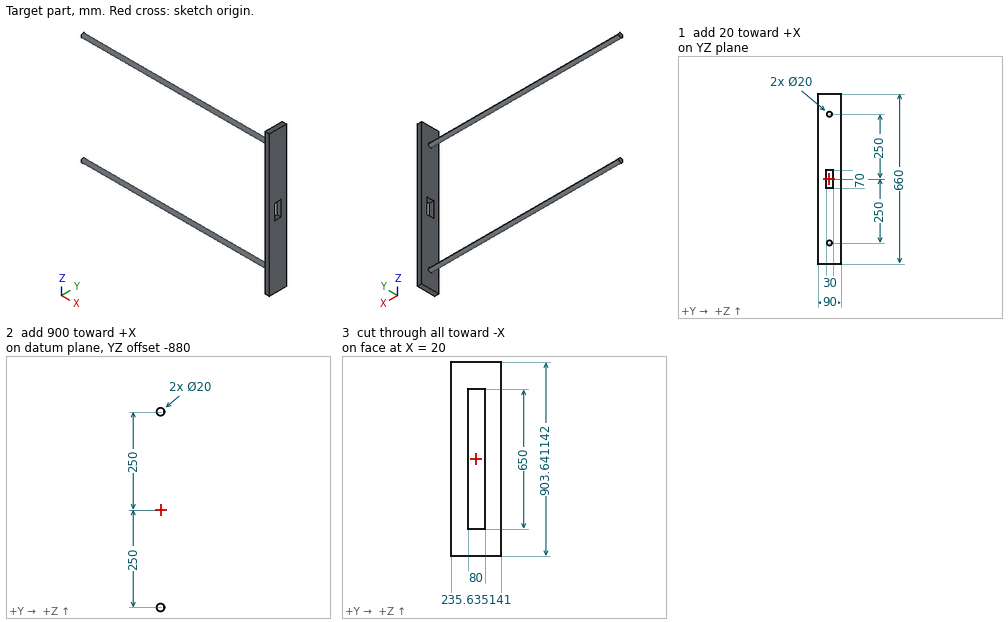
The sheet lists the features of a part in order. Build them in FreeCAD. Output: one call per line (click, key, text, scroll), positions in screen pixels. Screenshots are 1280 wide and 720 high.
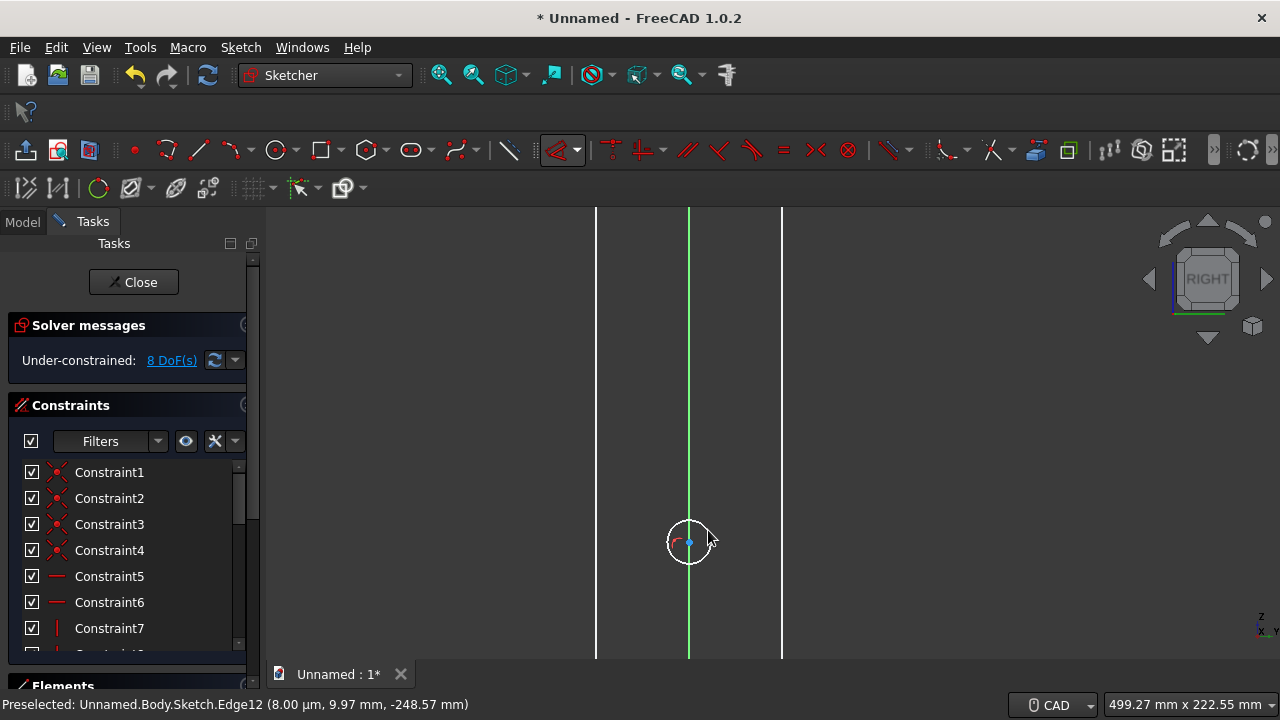
scroll(708, 535, down, 8)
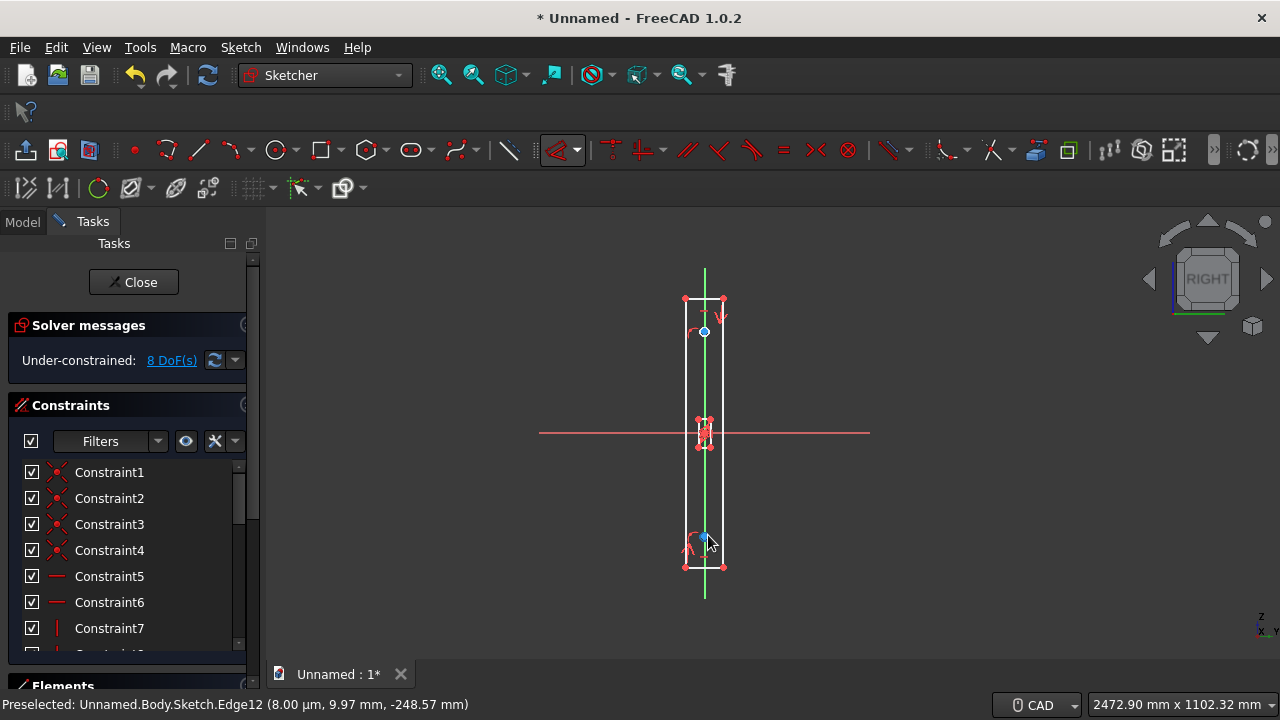
scroll(708, 329, up, 8)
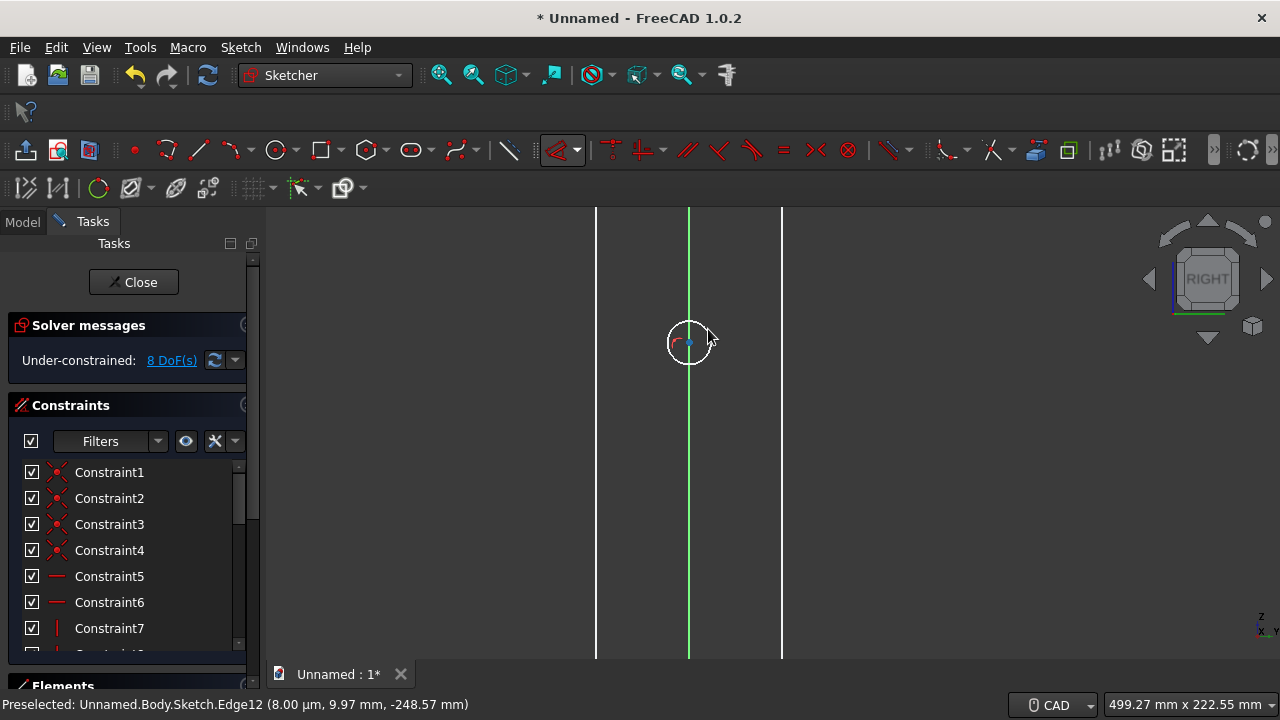
click(705, 327)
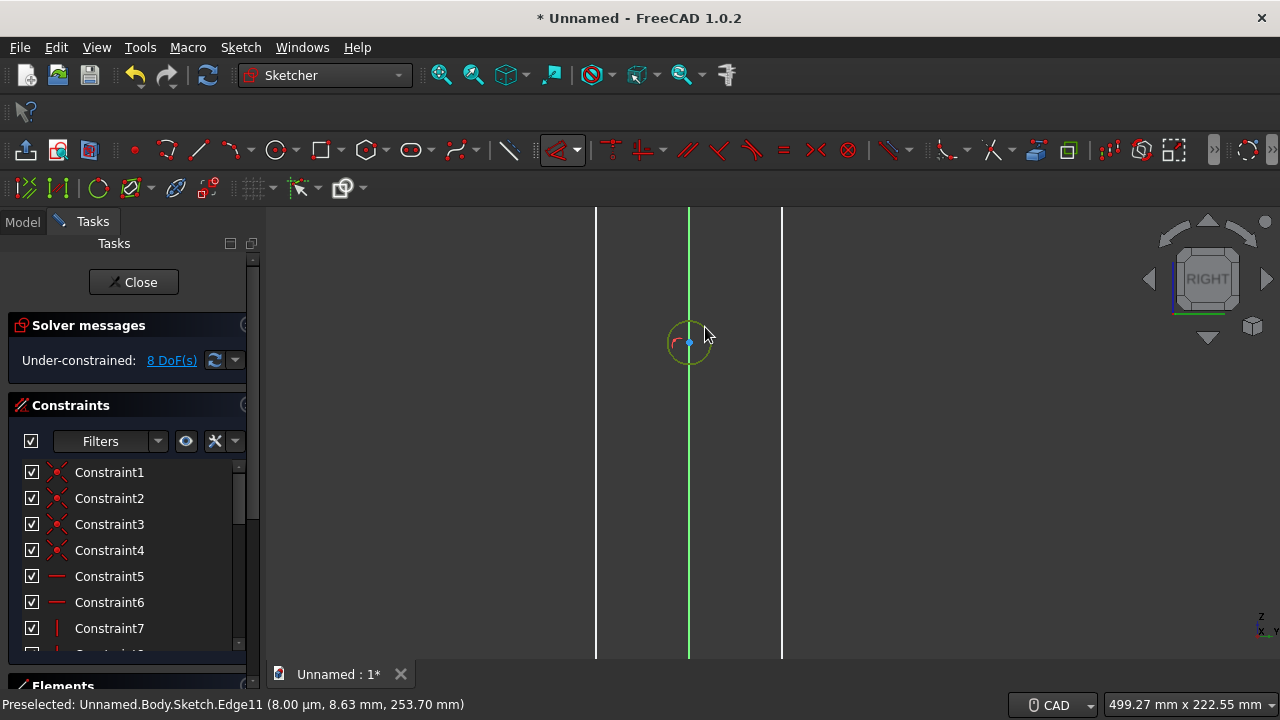
scroll(708, 329, down, 8)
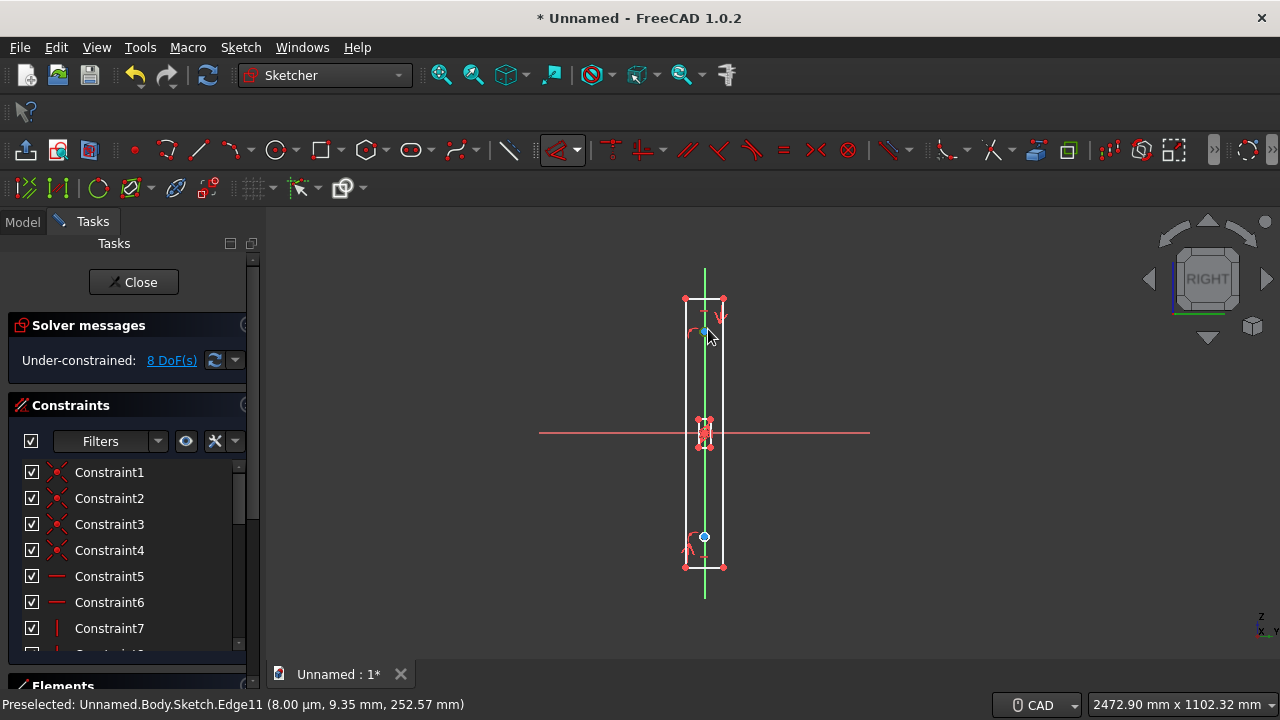
scroll(708, 534, up, 8)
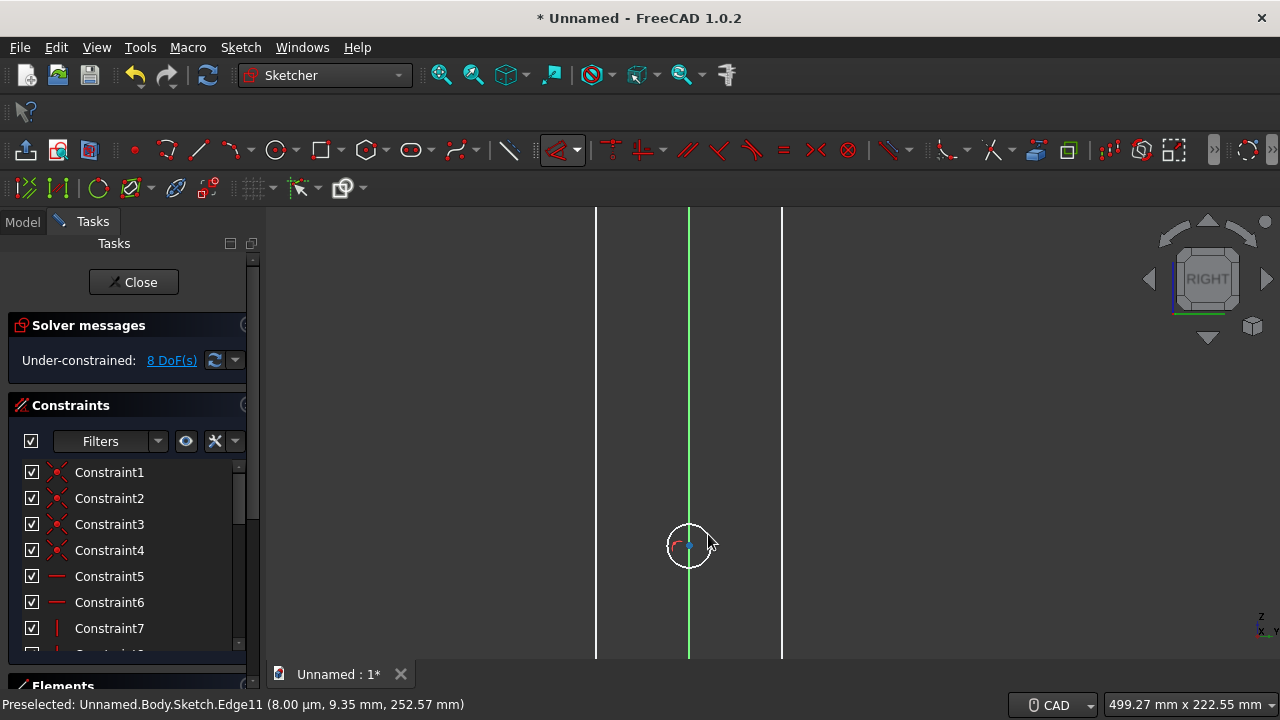
click(705, 531)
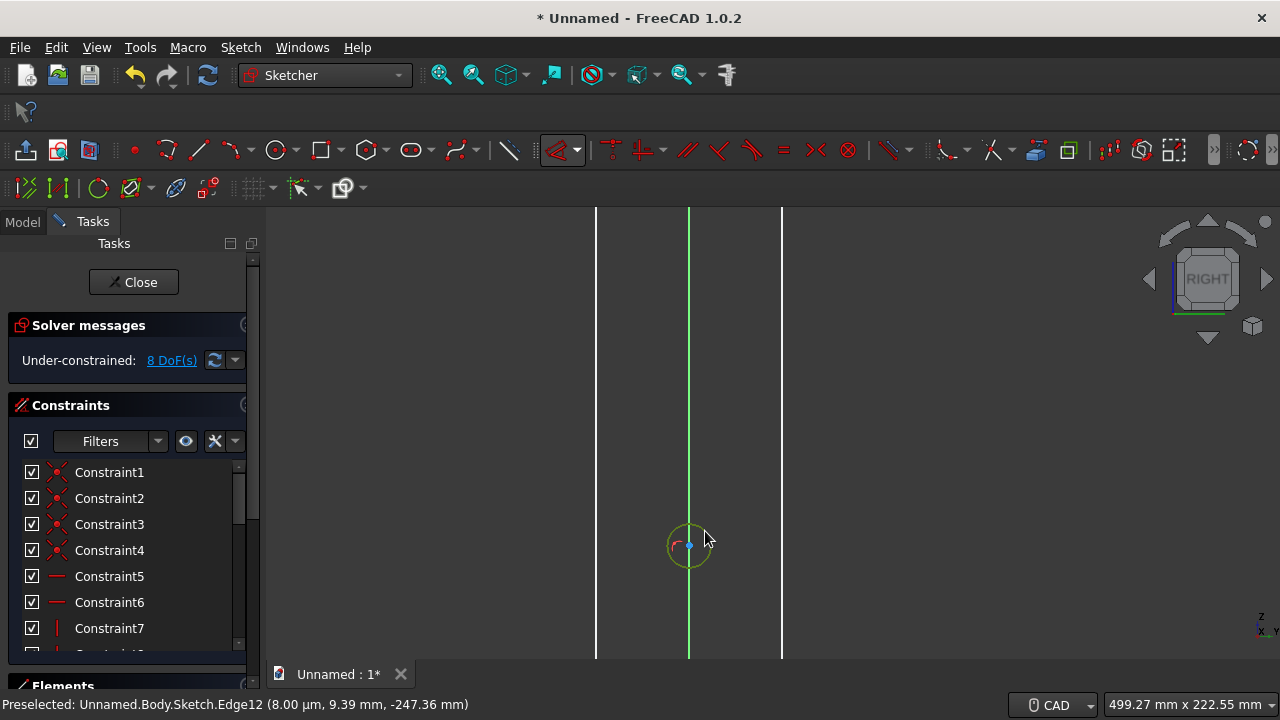
key(e)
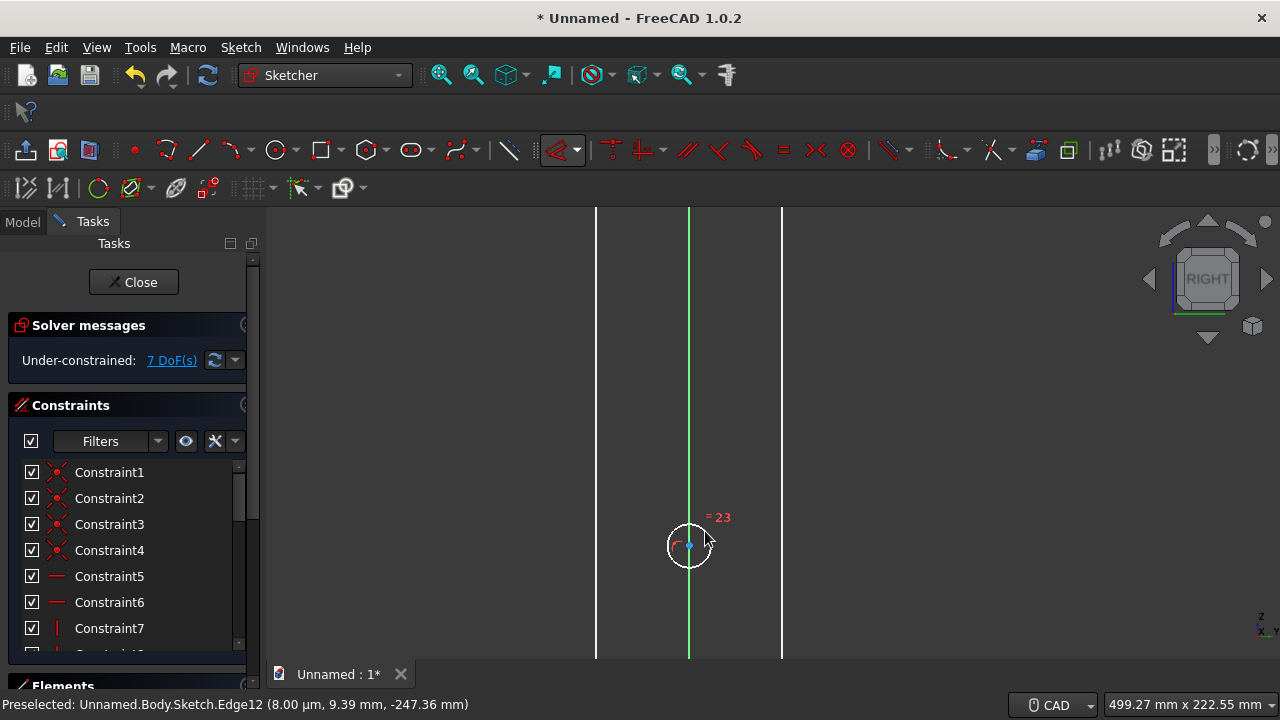
key(d)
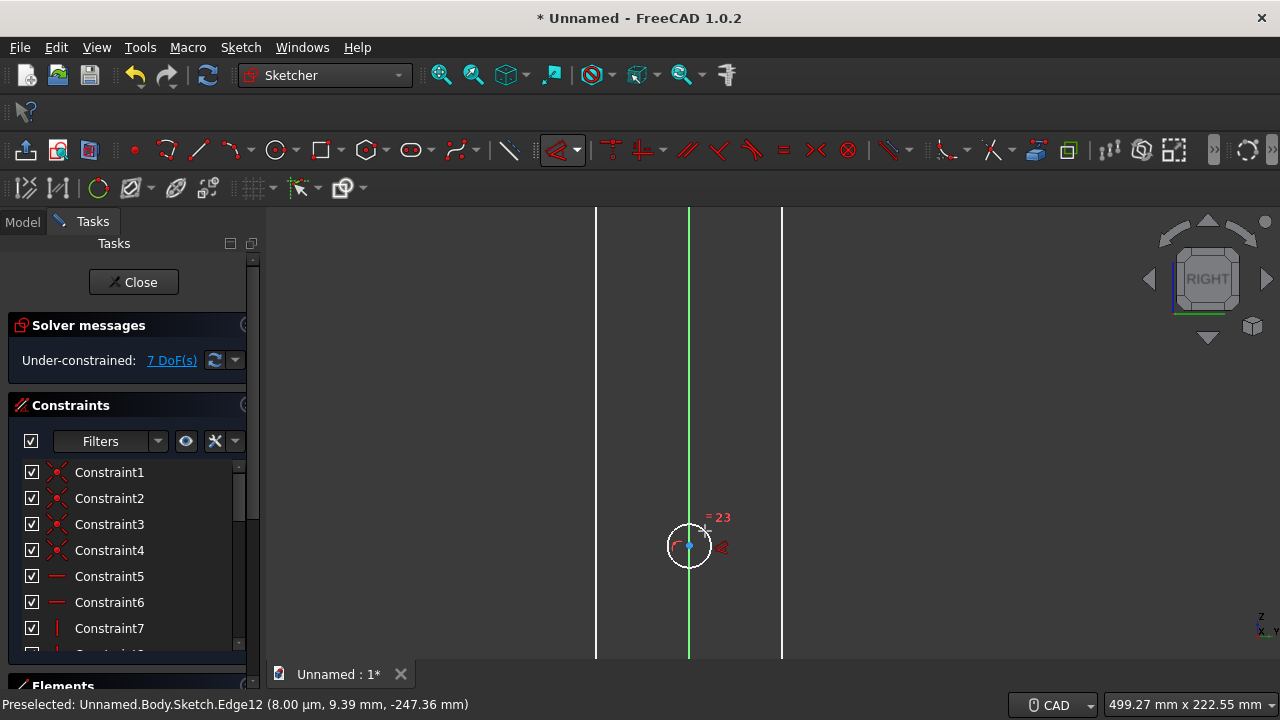
scroll(708, 534, down, 8)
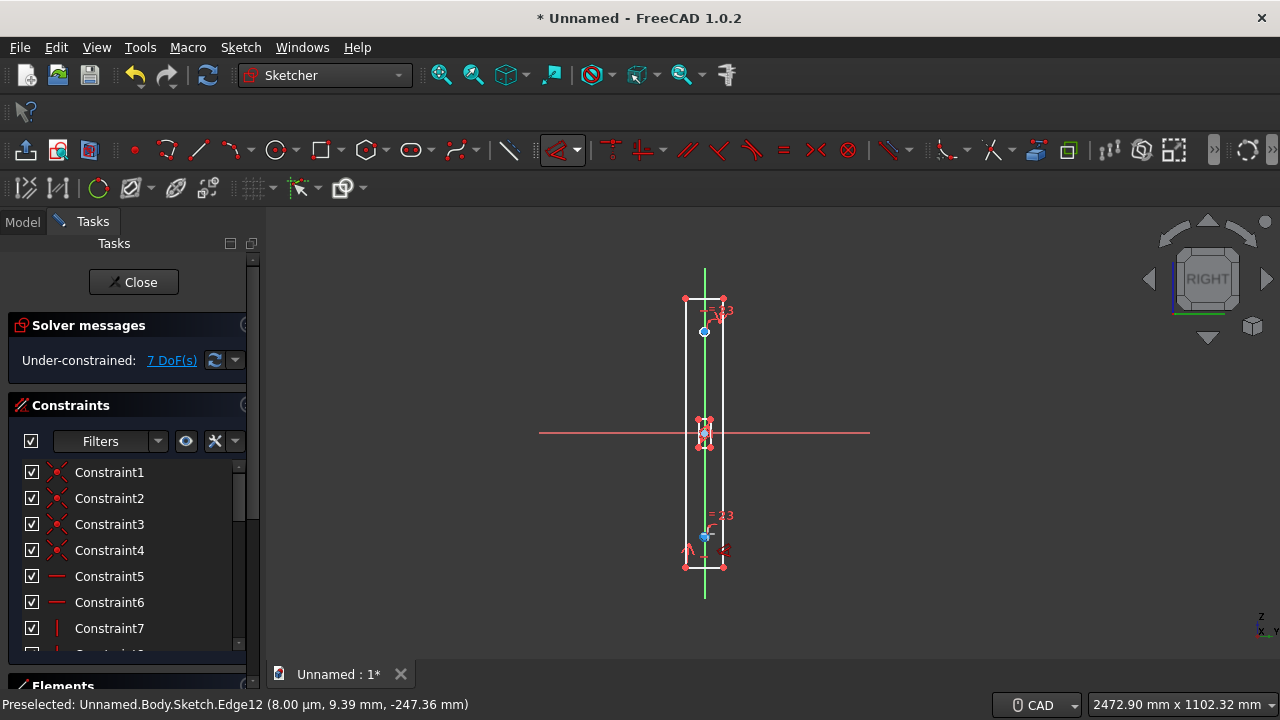
scroll(708, 329, up, 8)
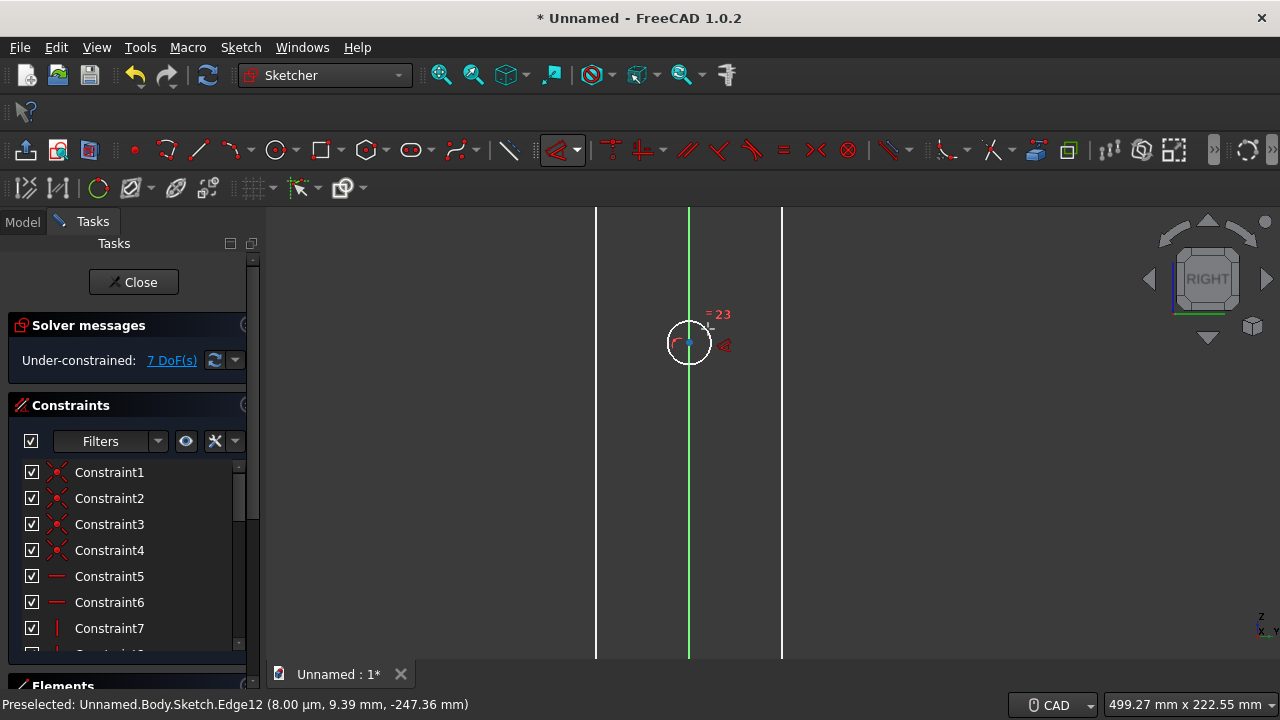
click(705, 327)
click(728, 304)